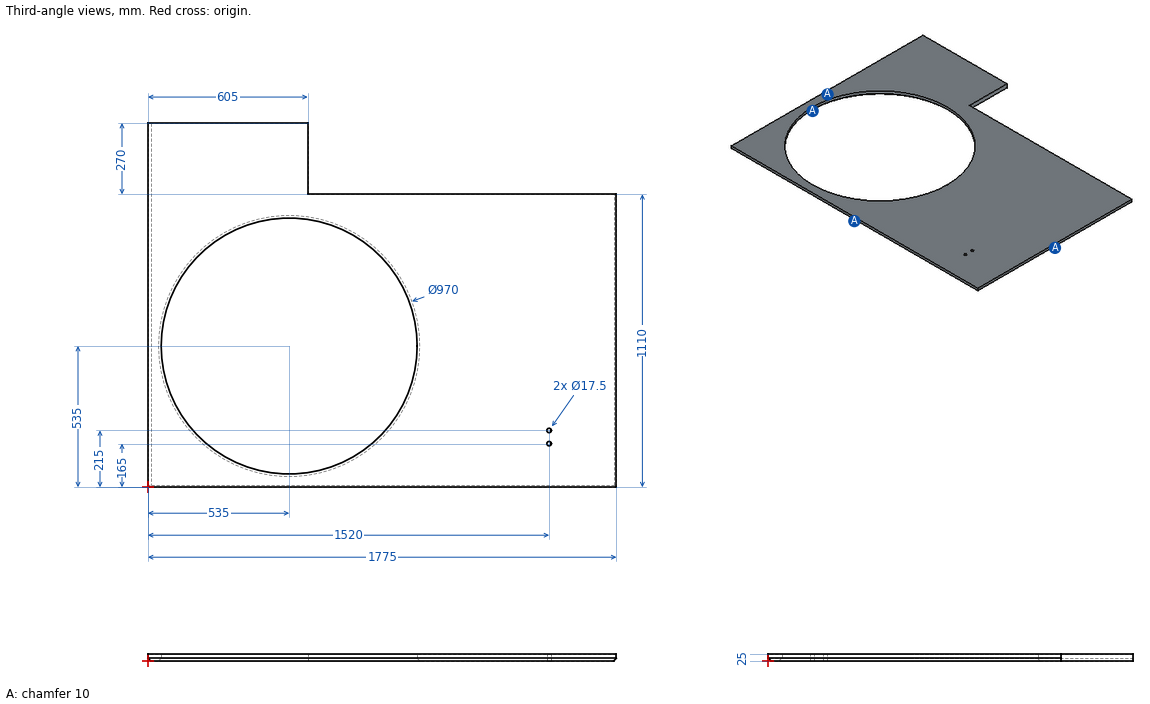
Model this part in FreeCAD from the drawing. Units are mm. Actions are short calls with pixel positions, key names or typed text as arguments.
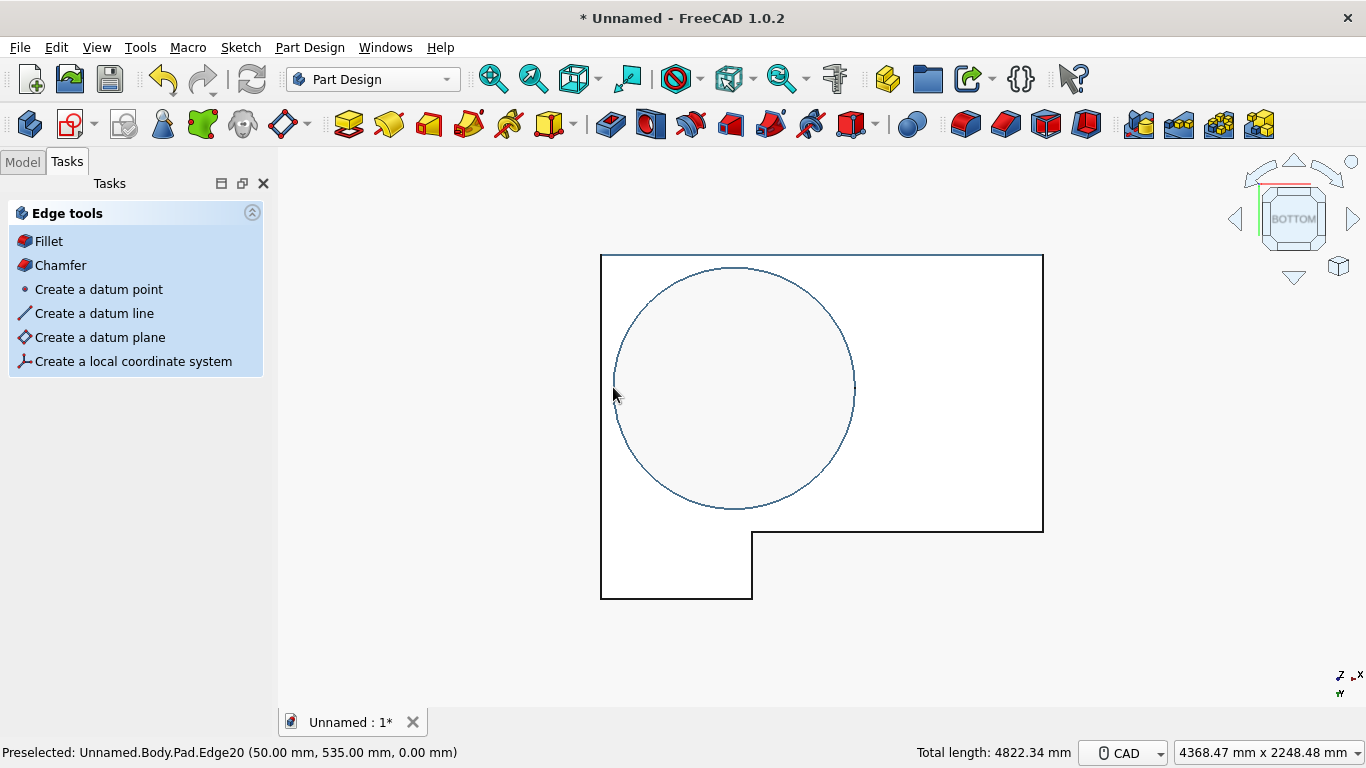
click(1043, 392, ctrl)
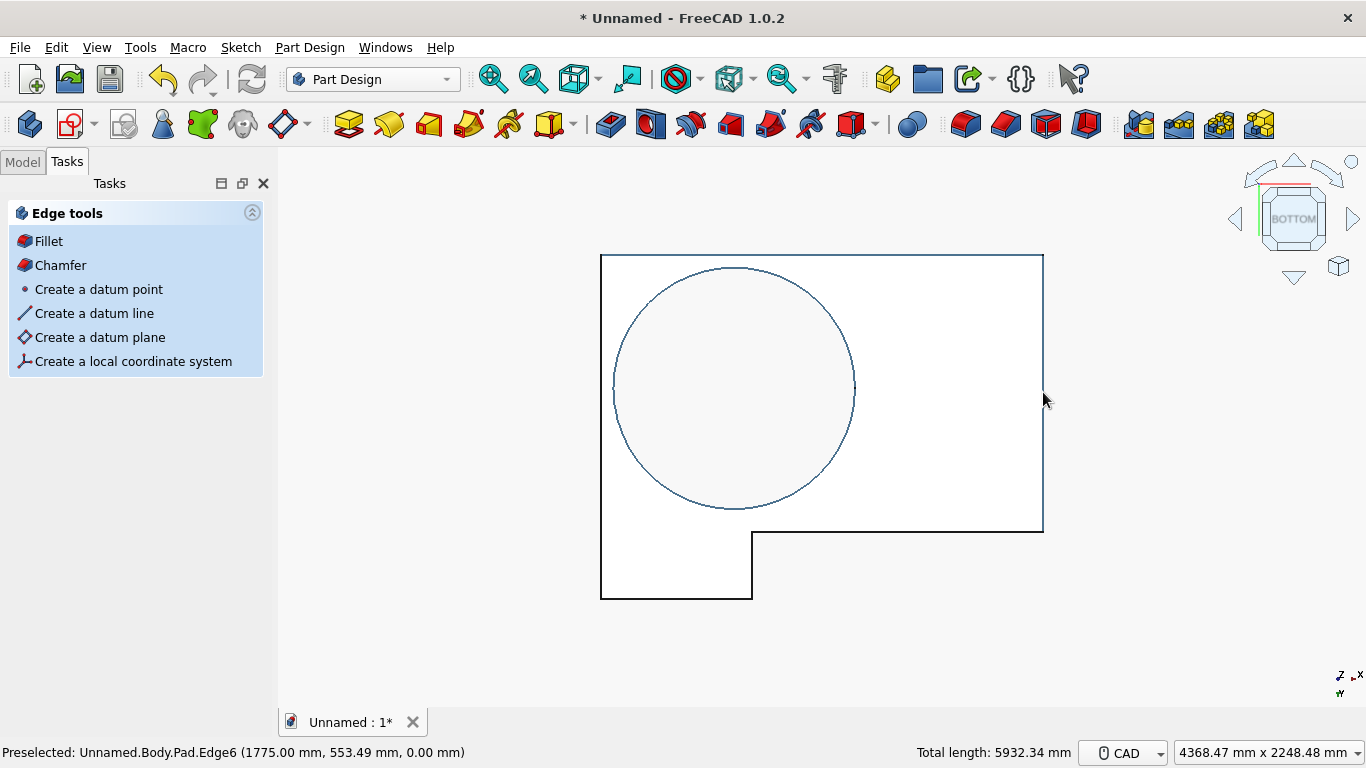
click(601, 426, ctrl)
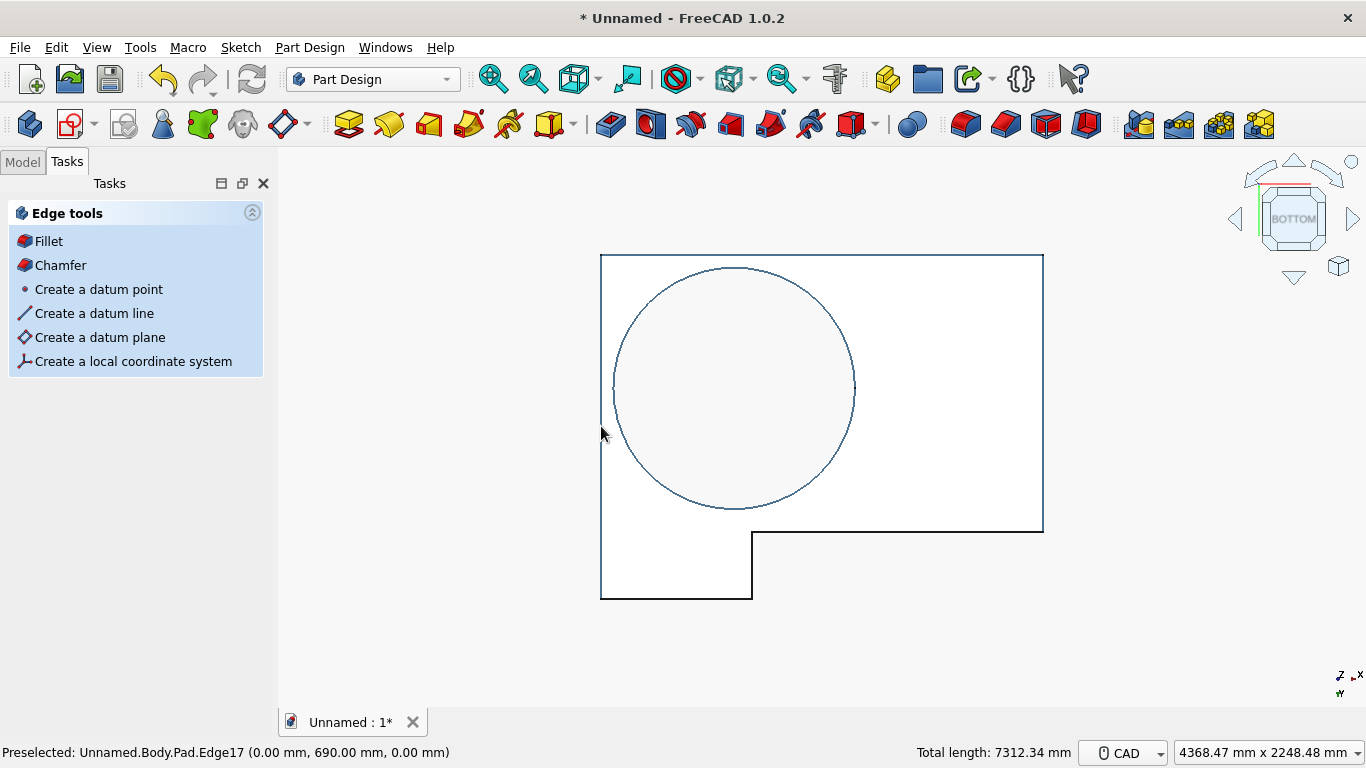
click(1006, 124)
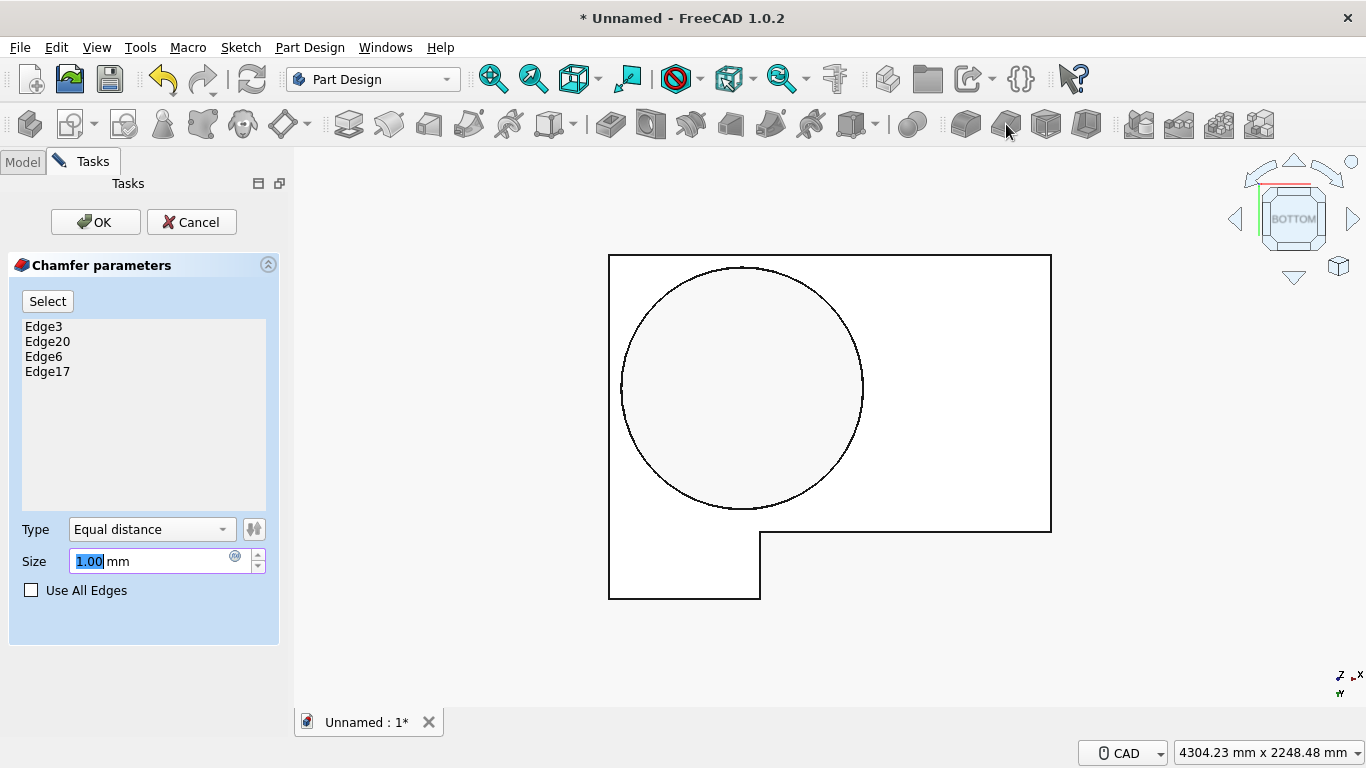
text(10)
key(Tab)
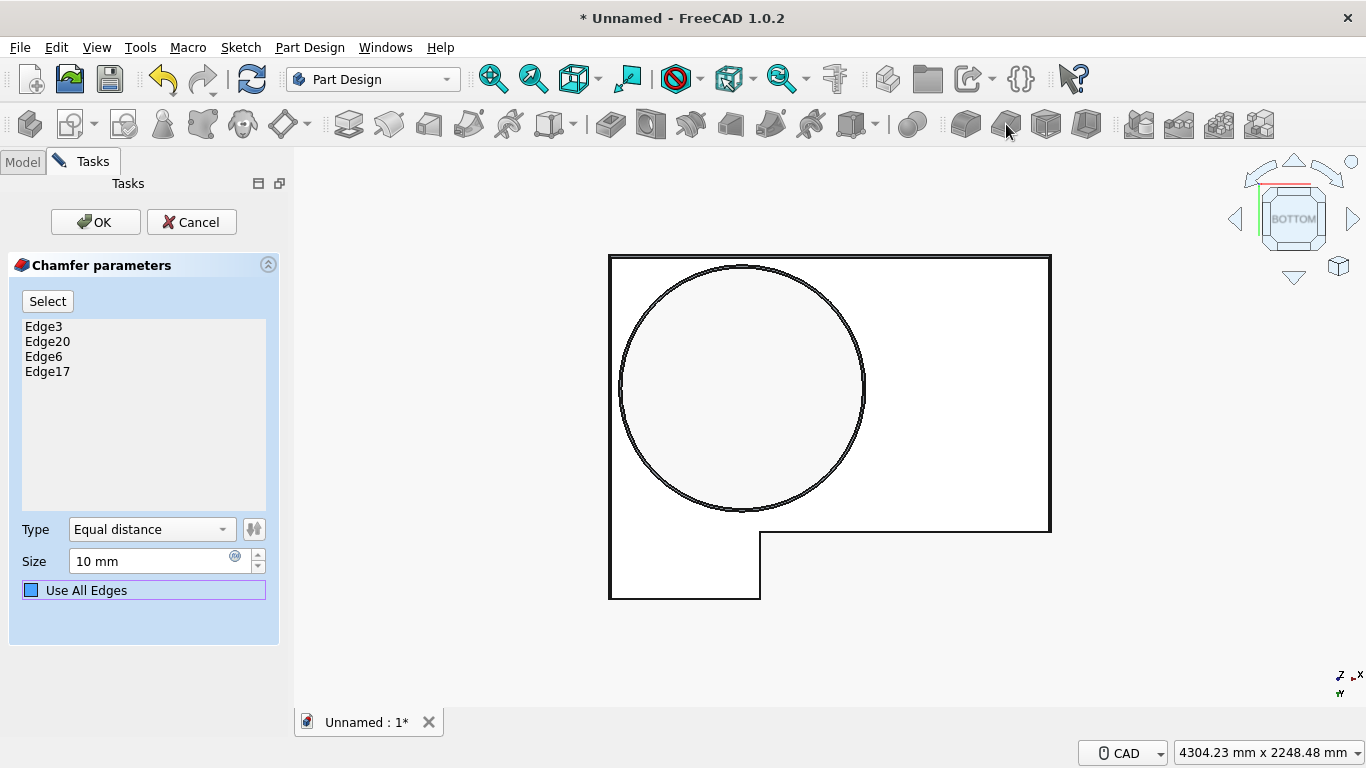
click(96, 222)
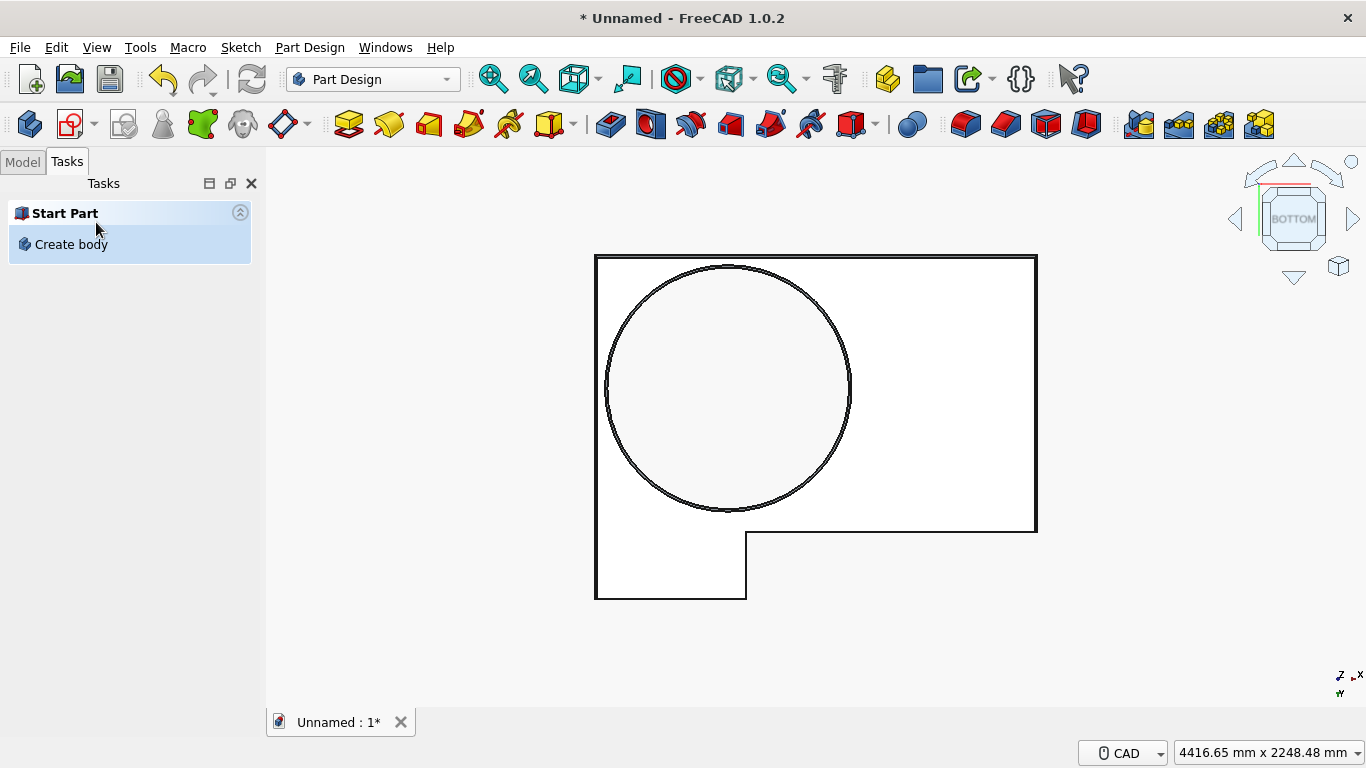
click(70, 124)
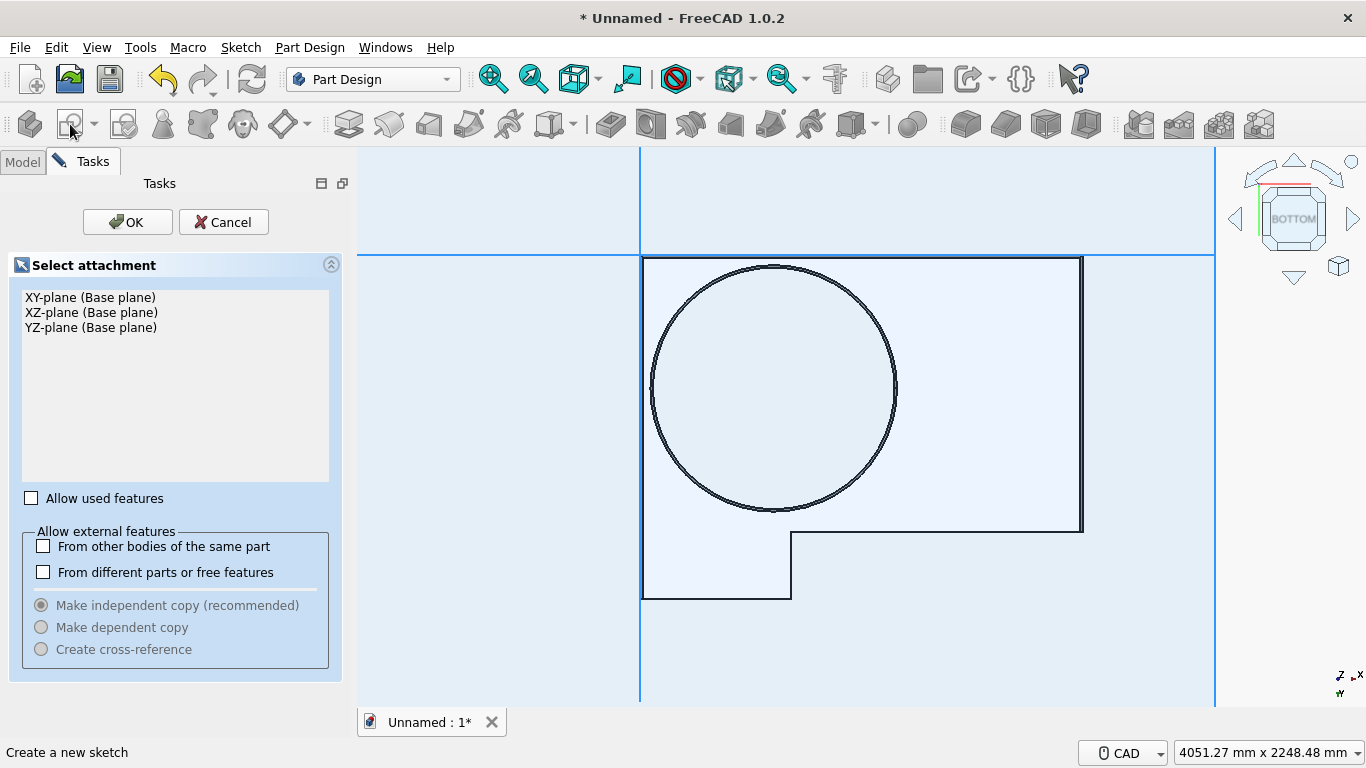
click(82, 298)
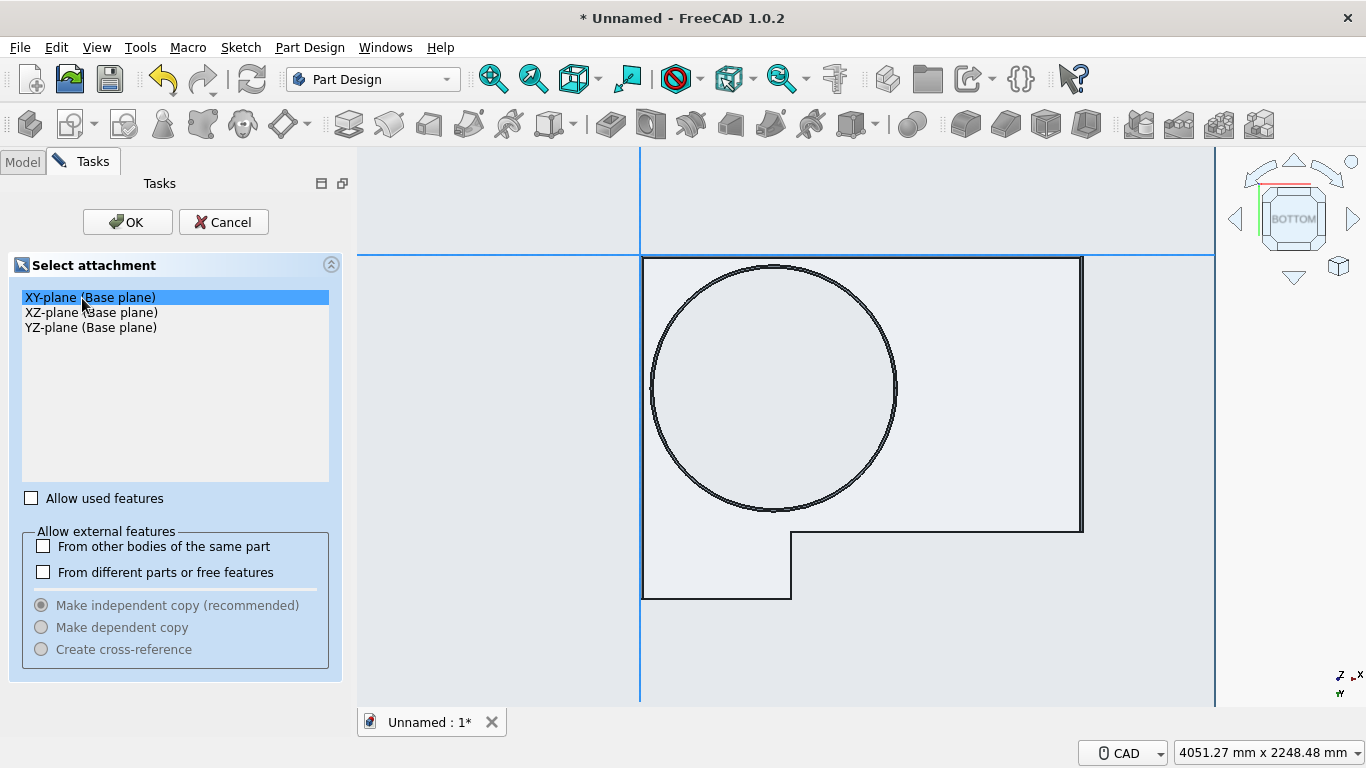
click(128, 222)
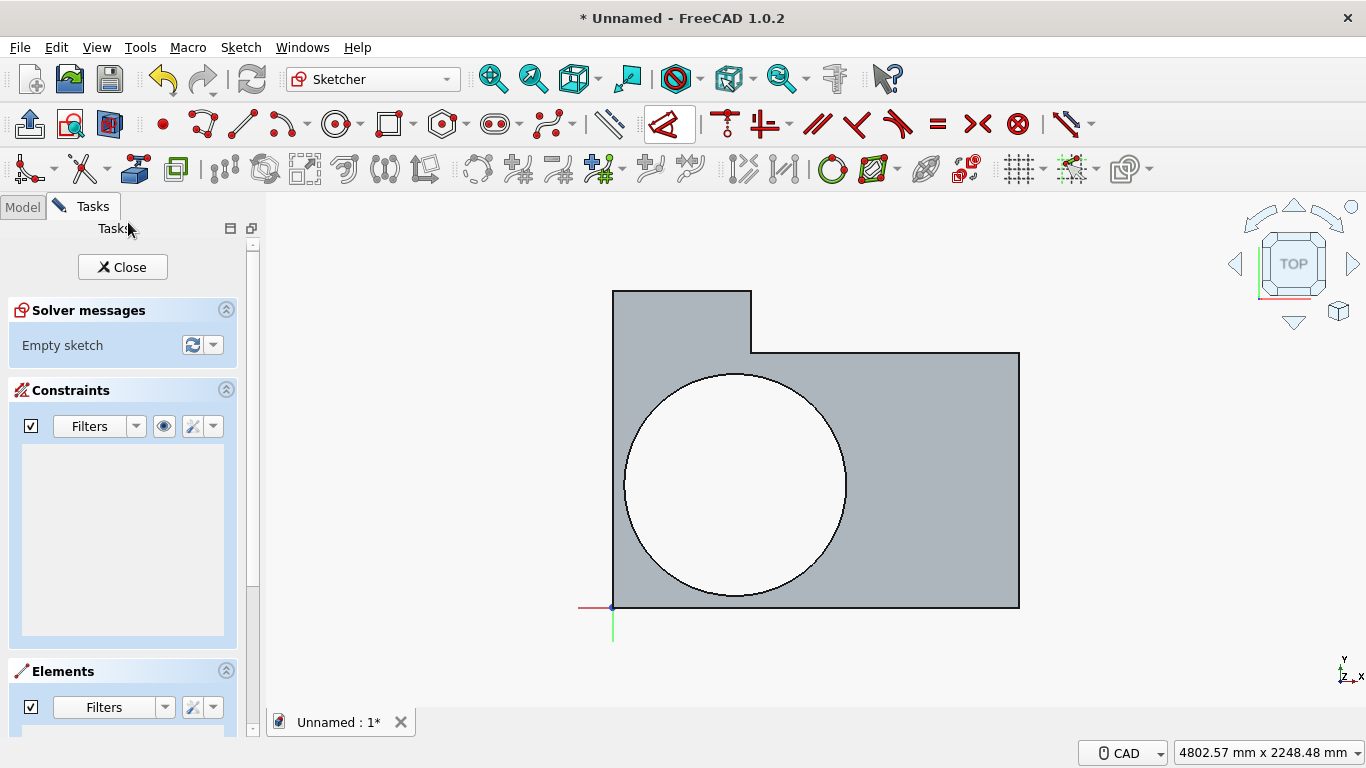
click(110, 124)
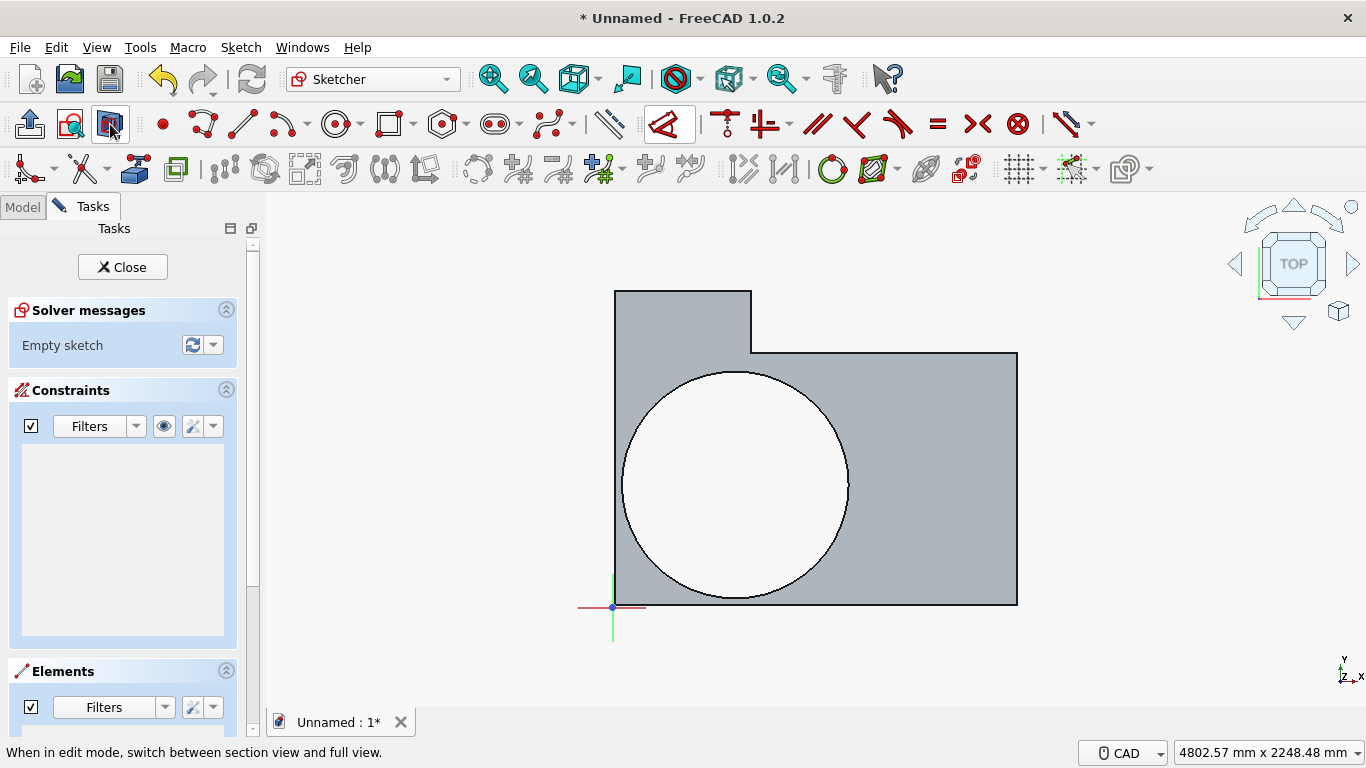
scroll(972, 570, up, 15)